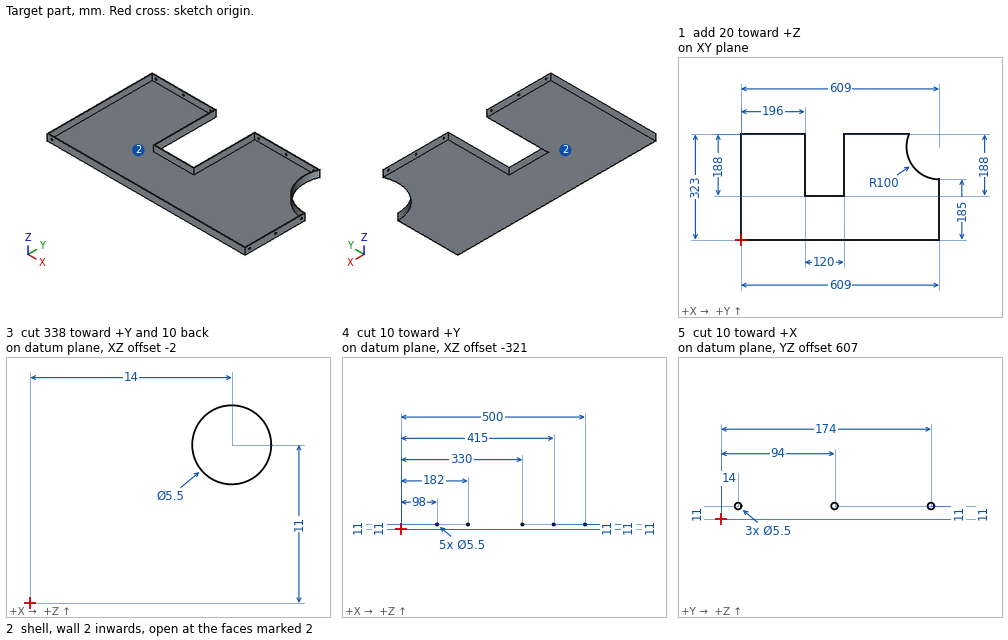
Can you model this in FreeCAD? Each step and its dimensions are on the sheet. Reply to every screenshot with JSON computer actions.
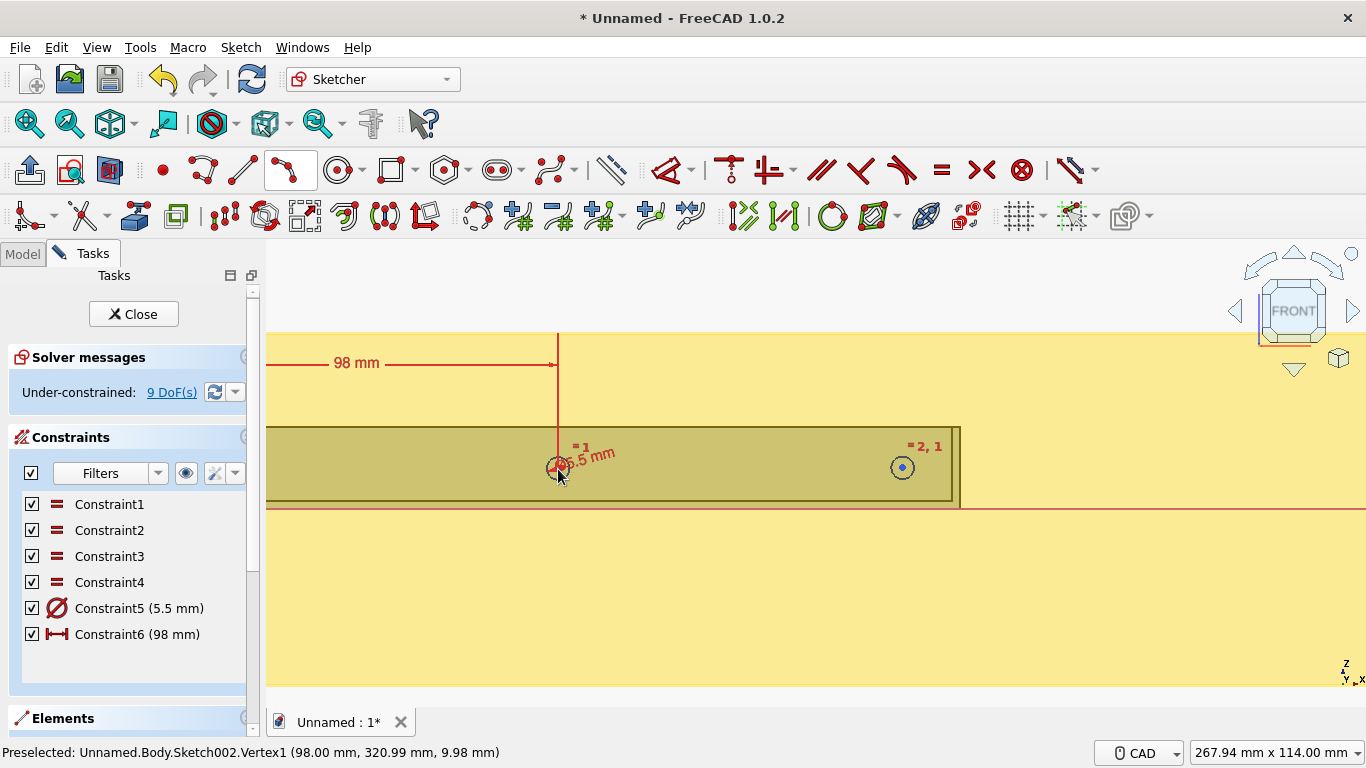
{"action": "left_click", "coordinate": [694, 170]}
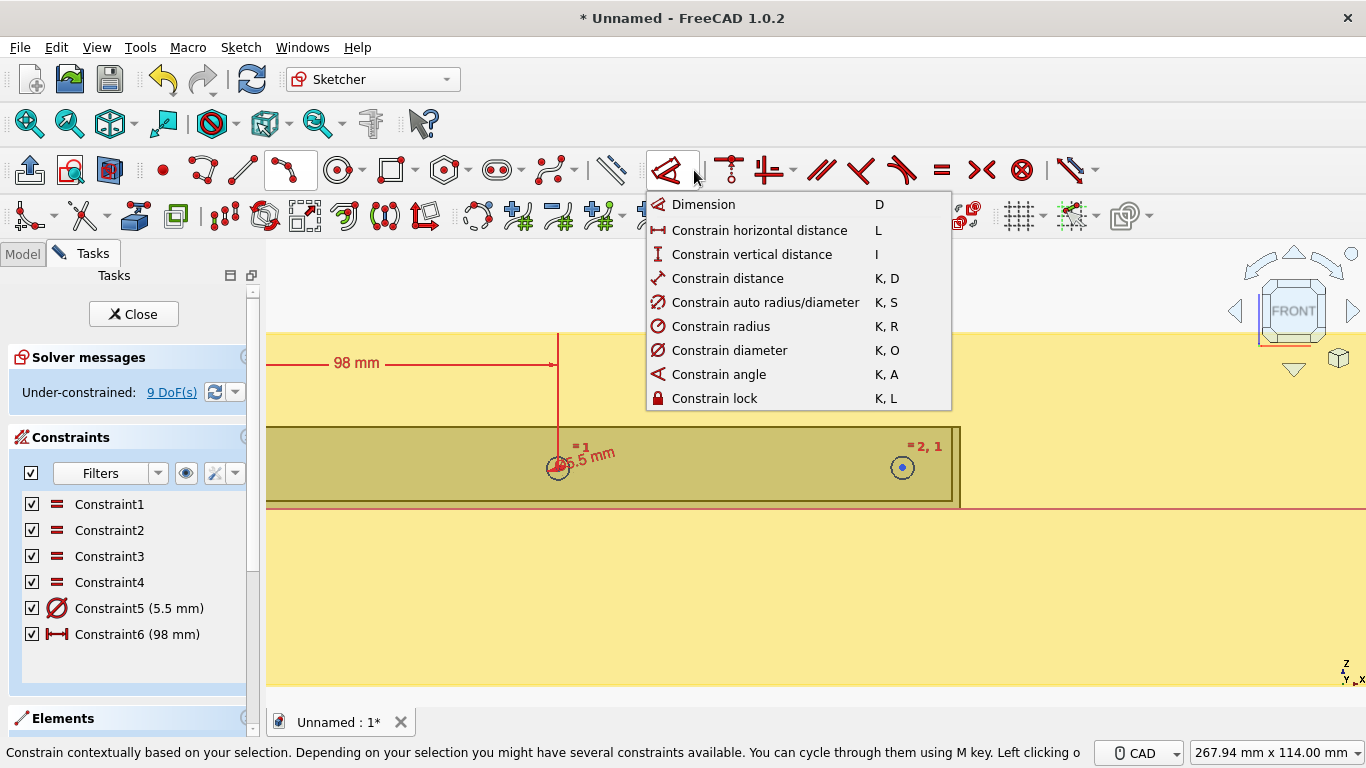
{"action": "left_click", "coordinate": [799, 254]}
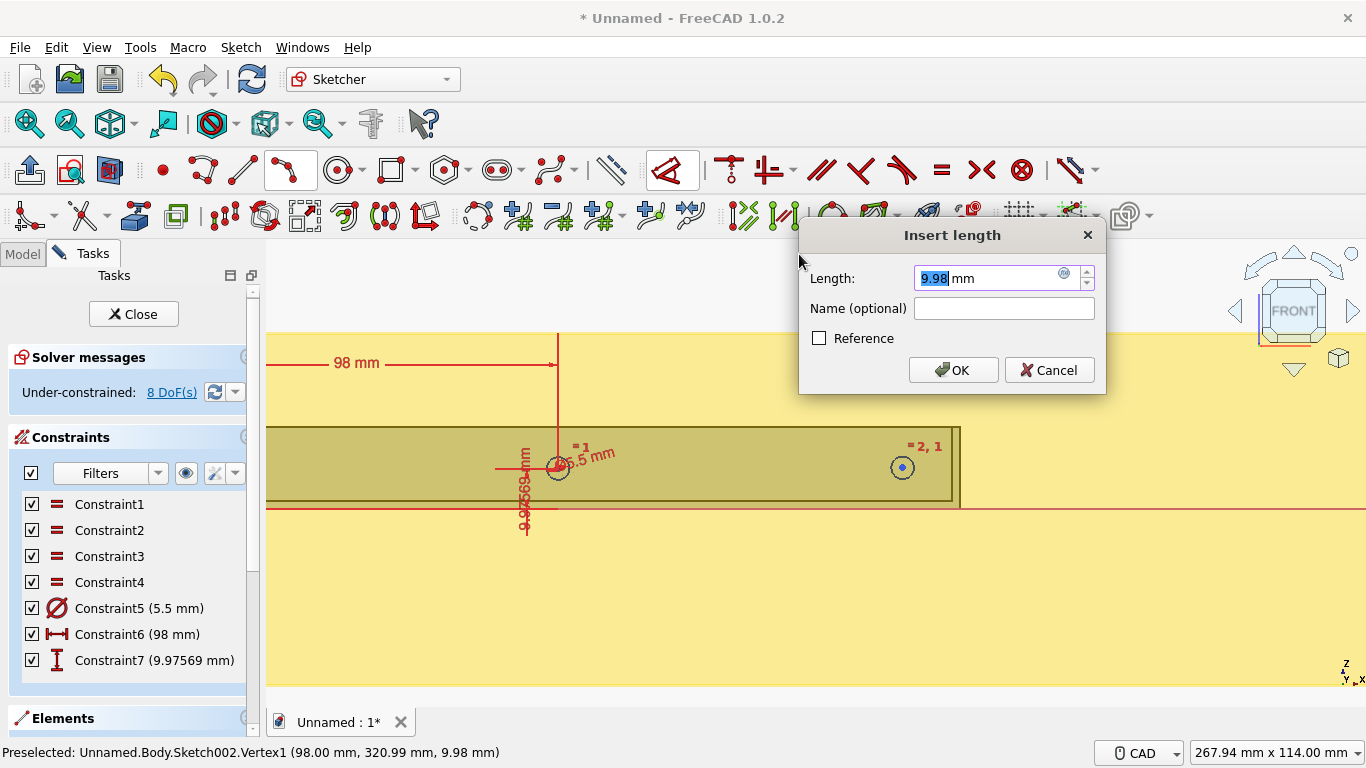
{"action": "type", "text": "11"}
{"action": "key", "text": "Return"}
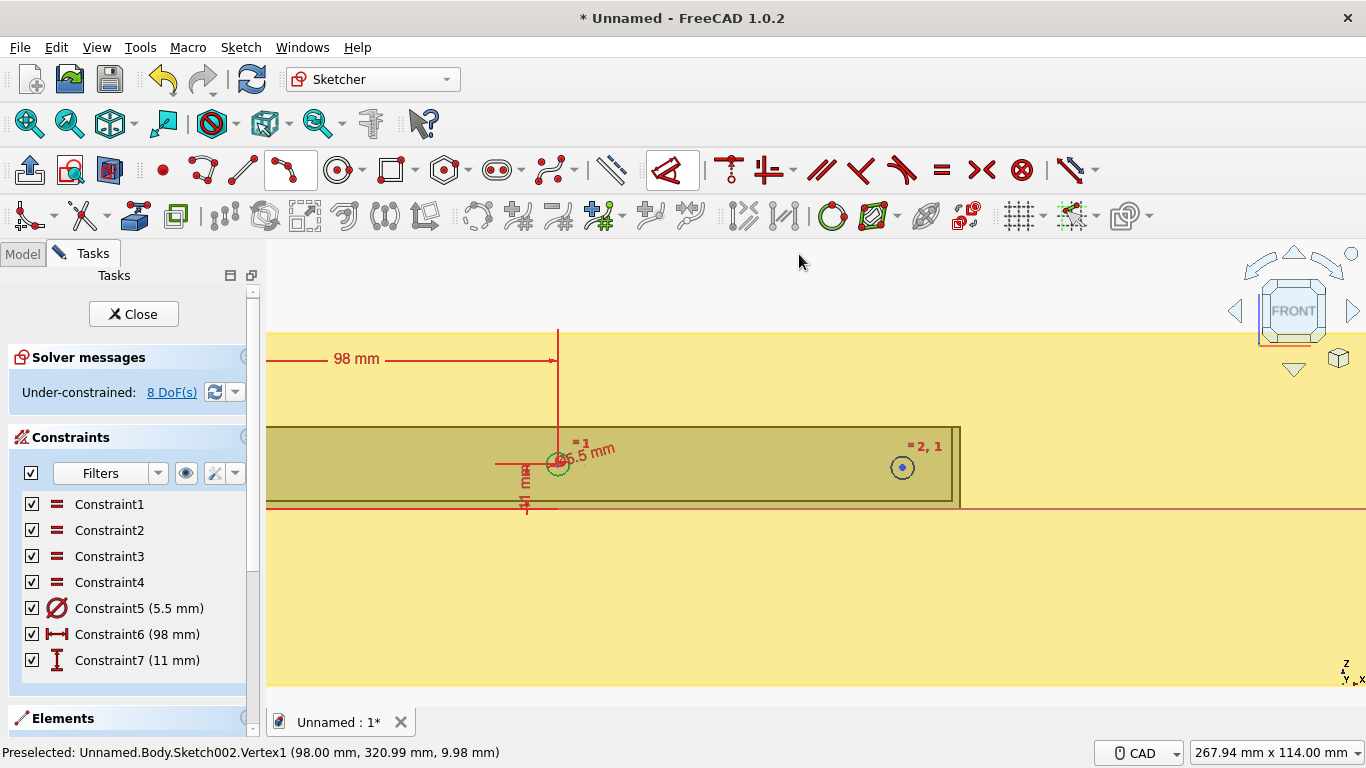
{"action": "left_click", "coordinate": [903, 468]}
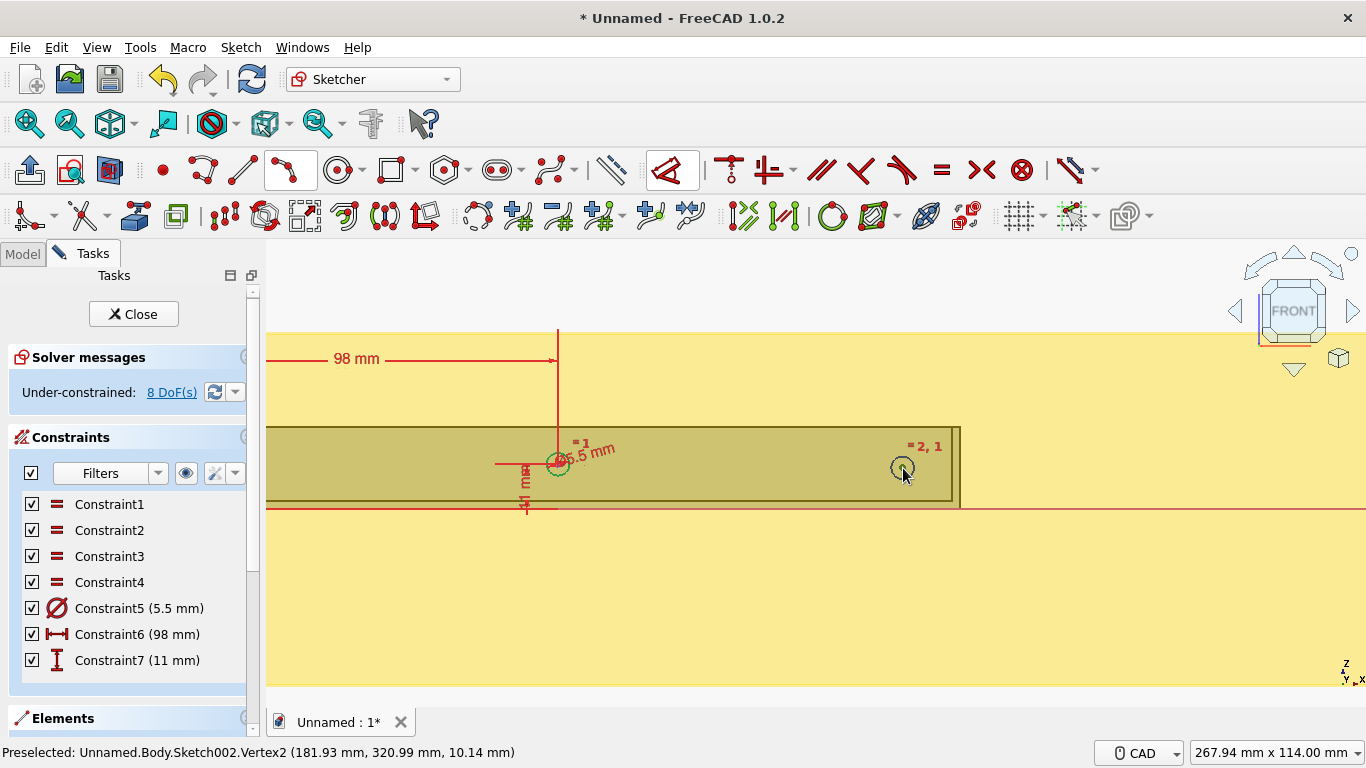
{"action": "key", "text": "i"}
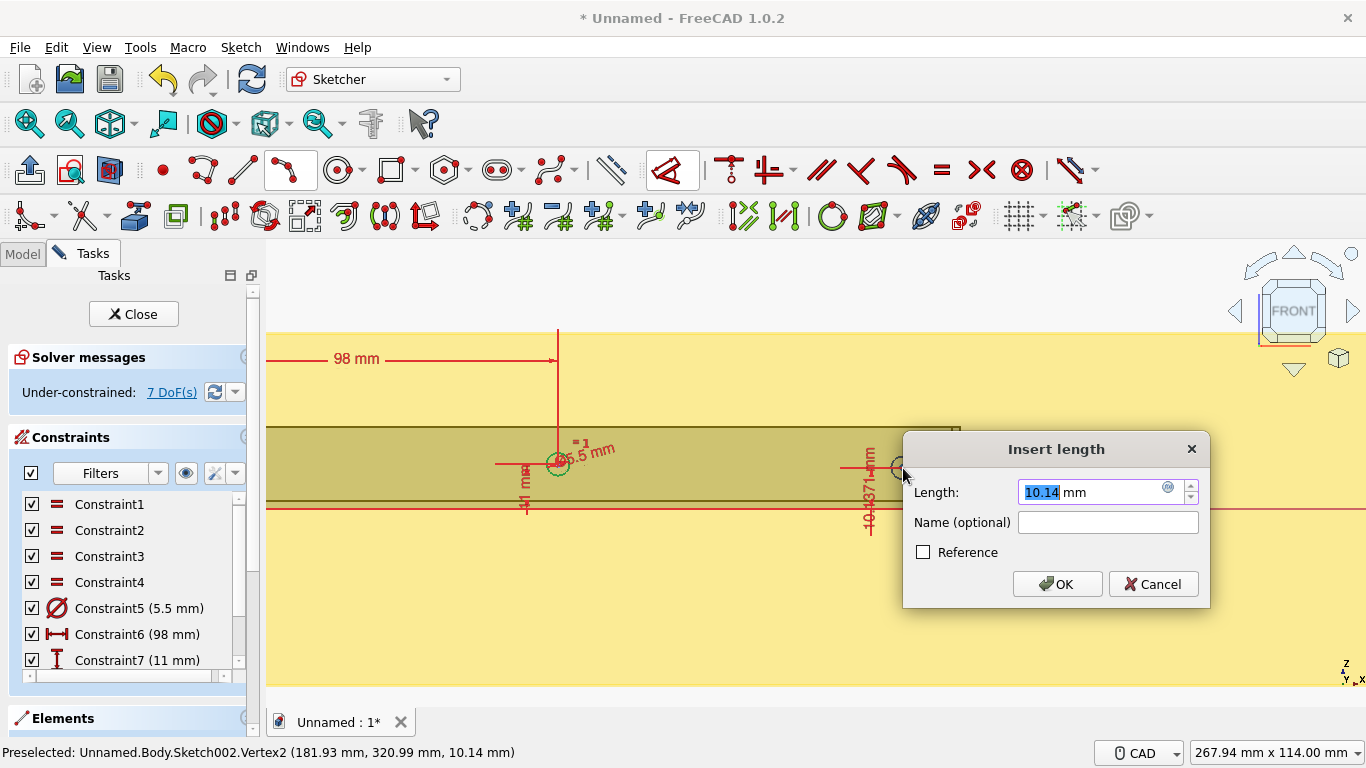
{"action": "type", "text": "11"}
{"action": "key", "text": "Return"}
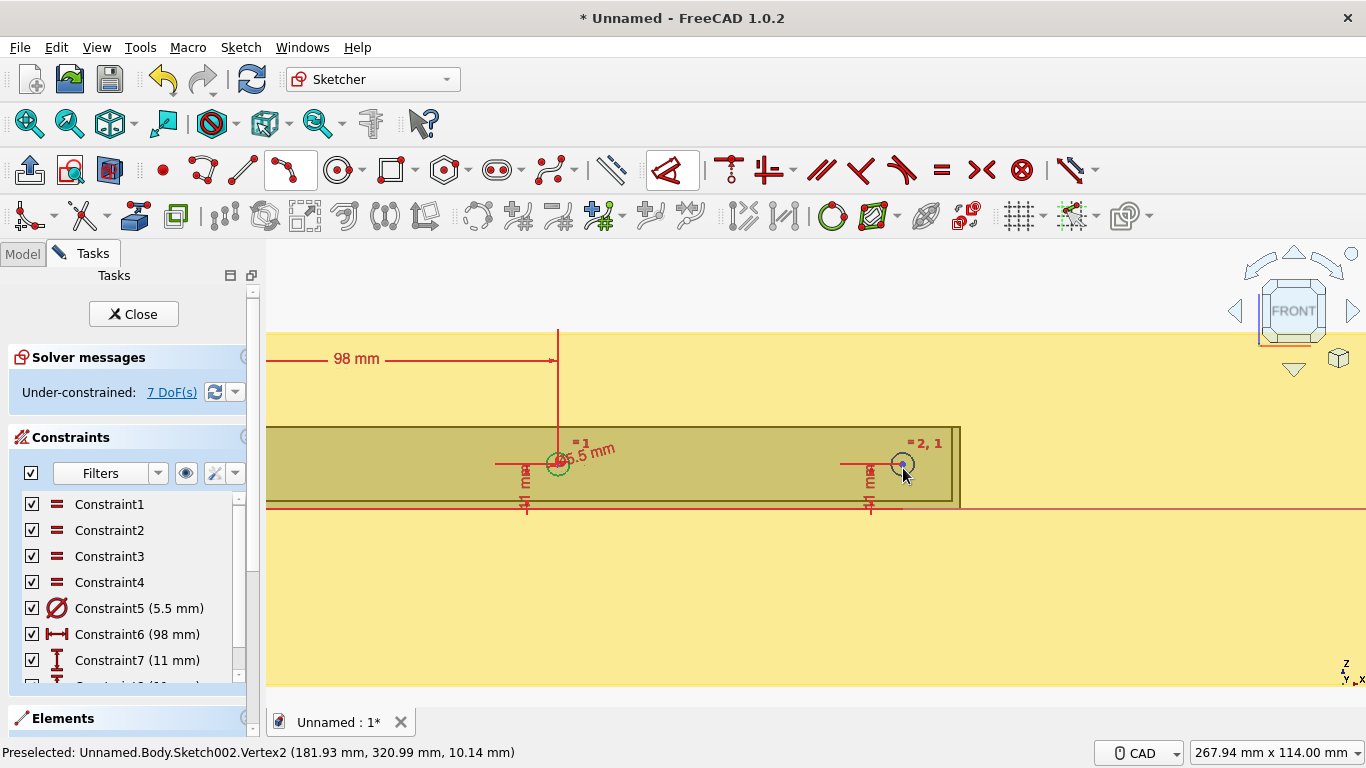
{"action": "scroll", "coordinate": [558, 469], "scroll_direction": "down", "scroll_amount": 6}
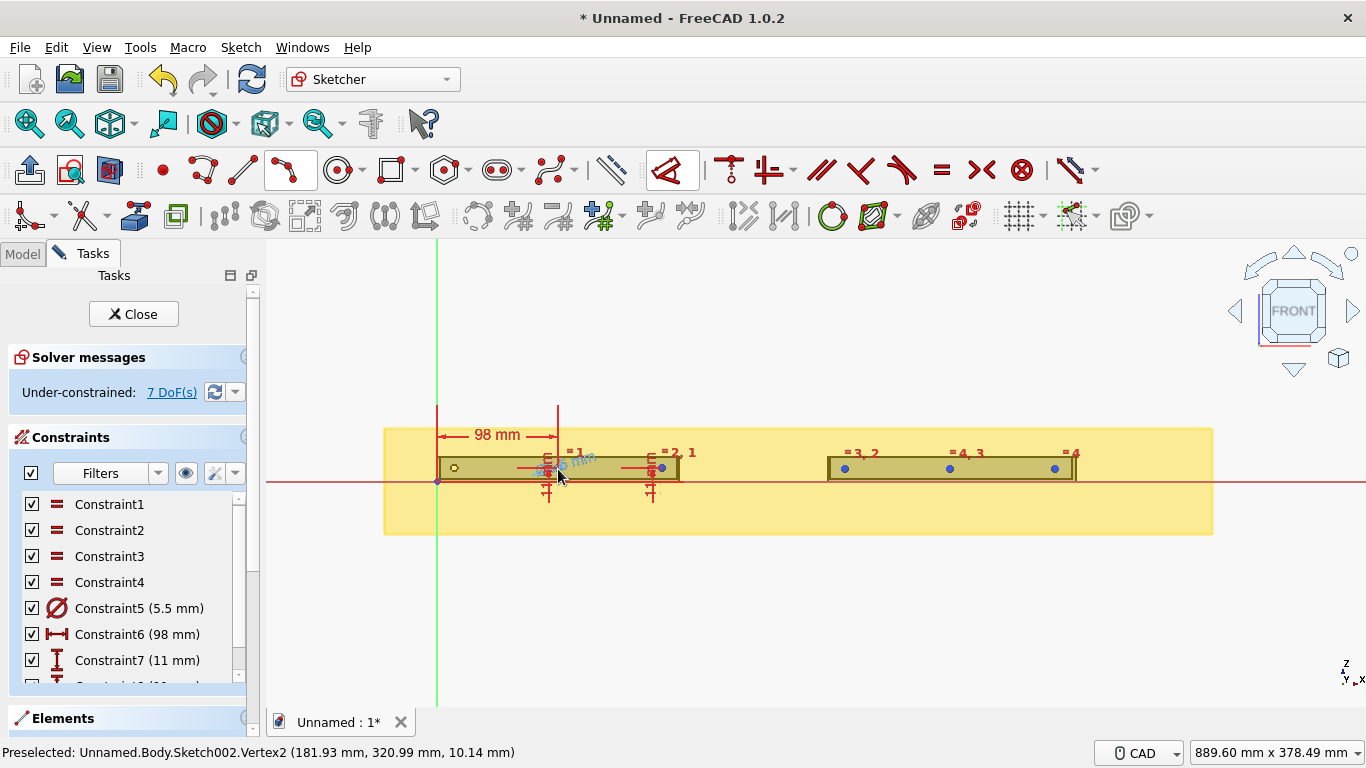
{"action": "scroll", "coordinate": [845, 469], "scroll_direction": "up", "scroll_amount": 6}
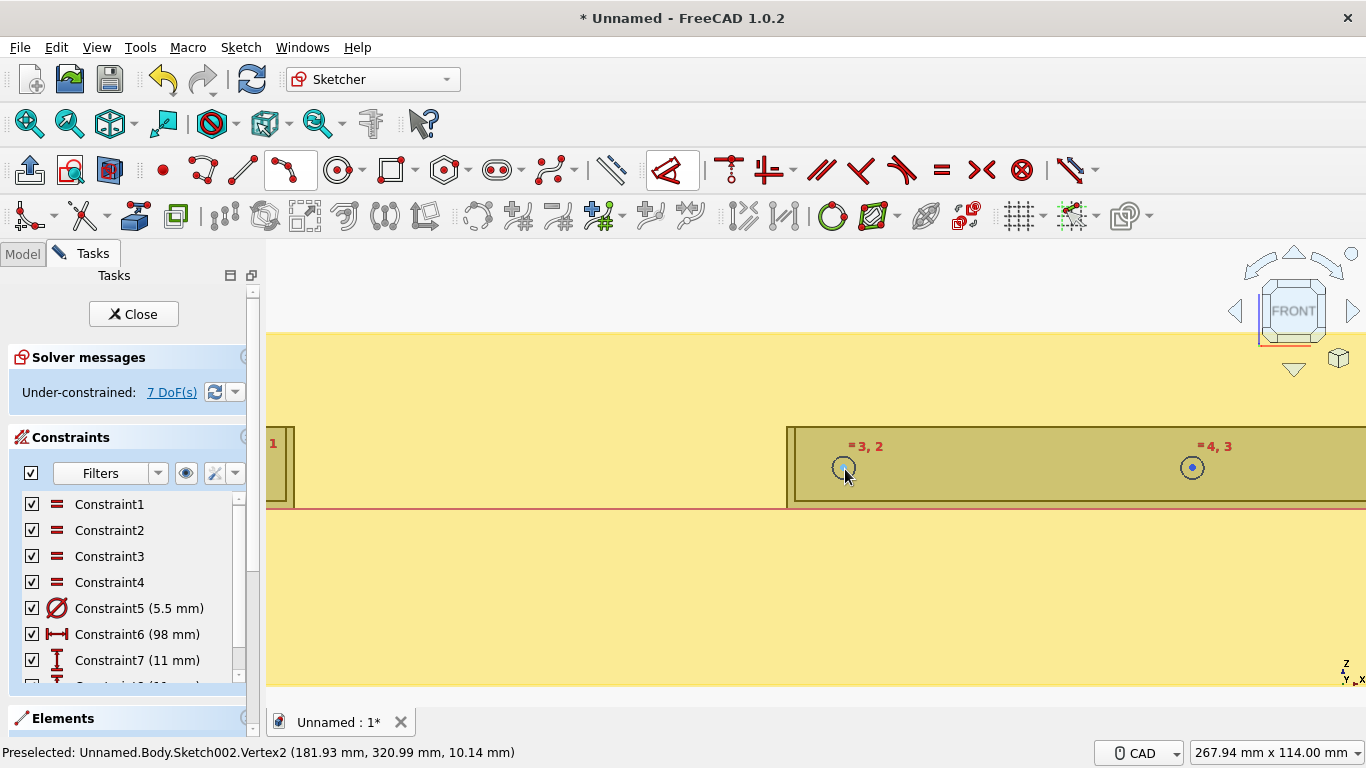
{"action": "left_click", "coordinate": [844, 468]}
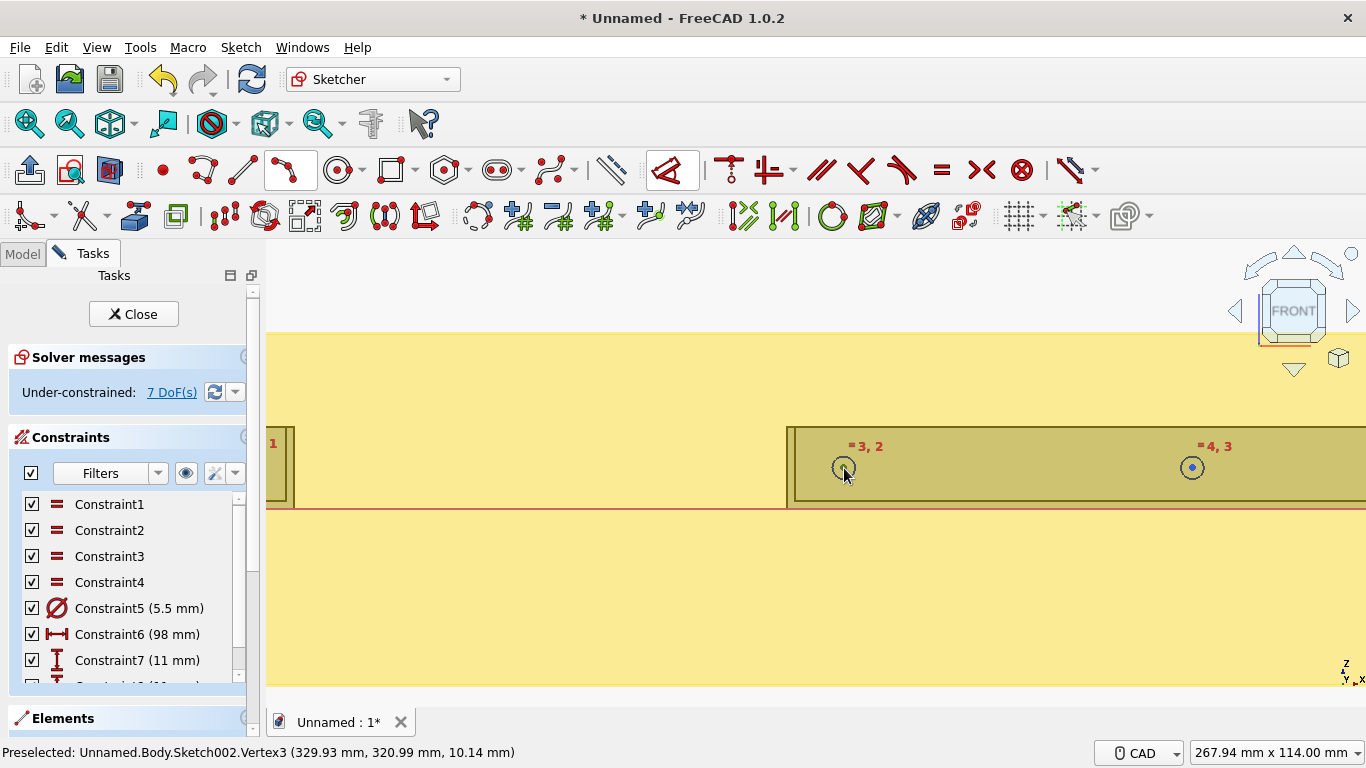
{"action": "key", "text": "i"}